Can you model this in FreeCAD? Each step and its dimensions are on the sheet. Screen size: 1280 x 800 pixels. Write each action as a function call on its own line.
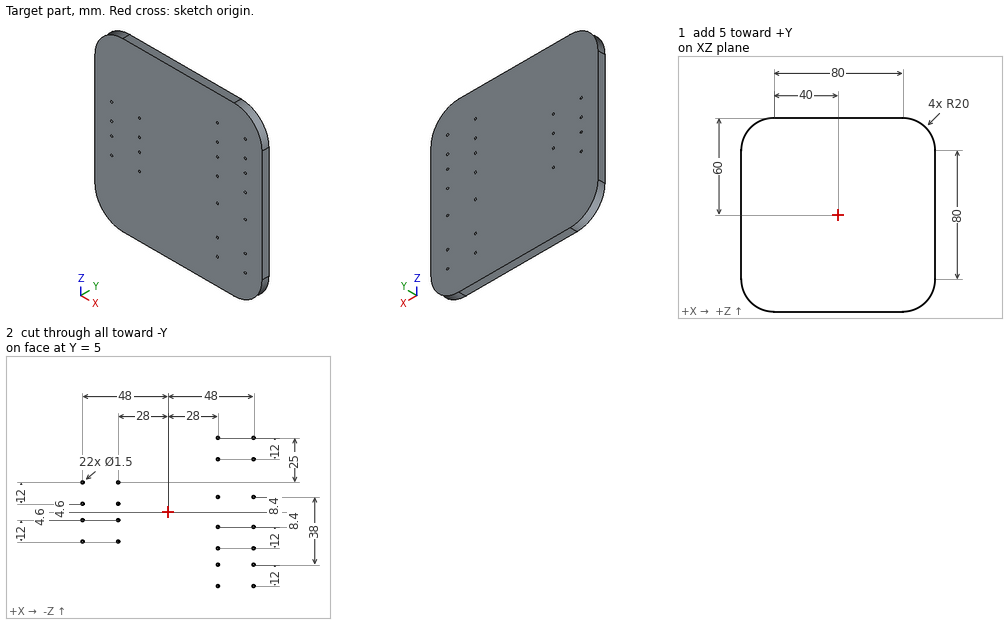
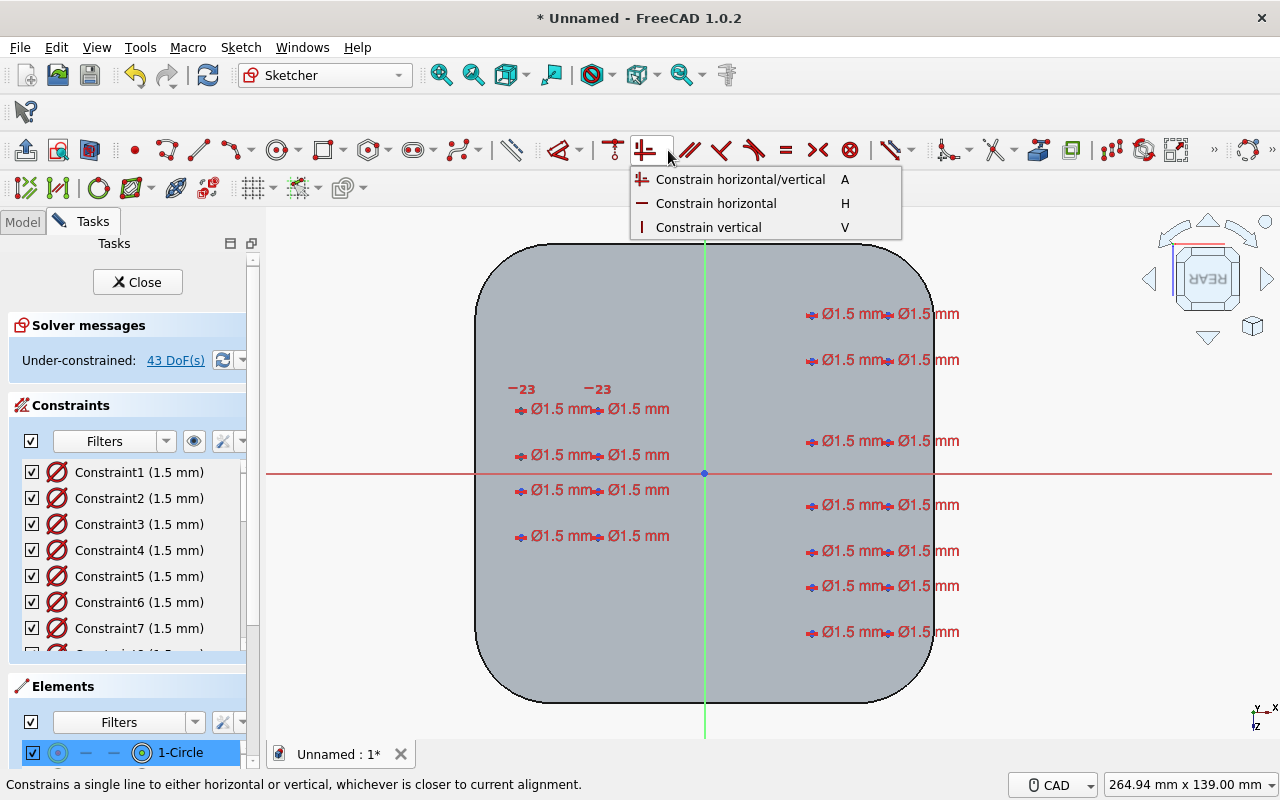
click(766, 227)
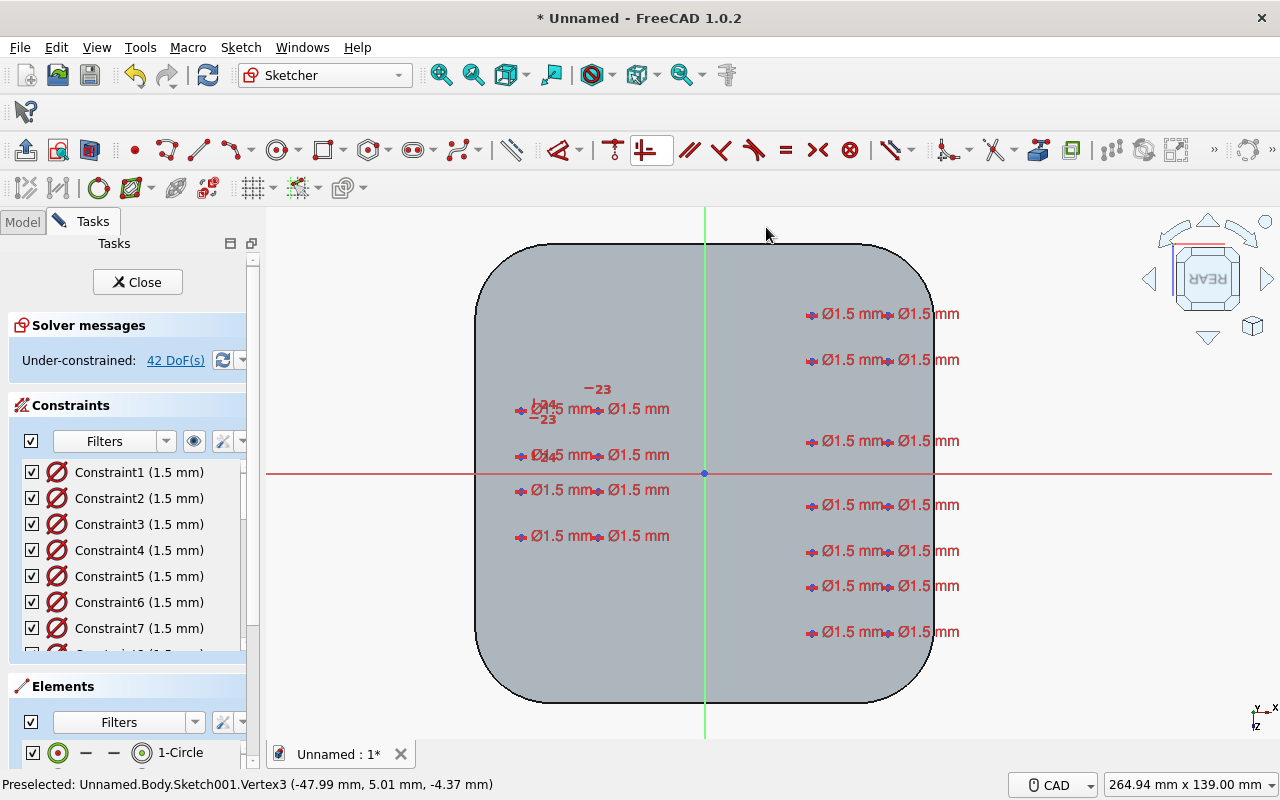
click(598, 411)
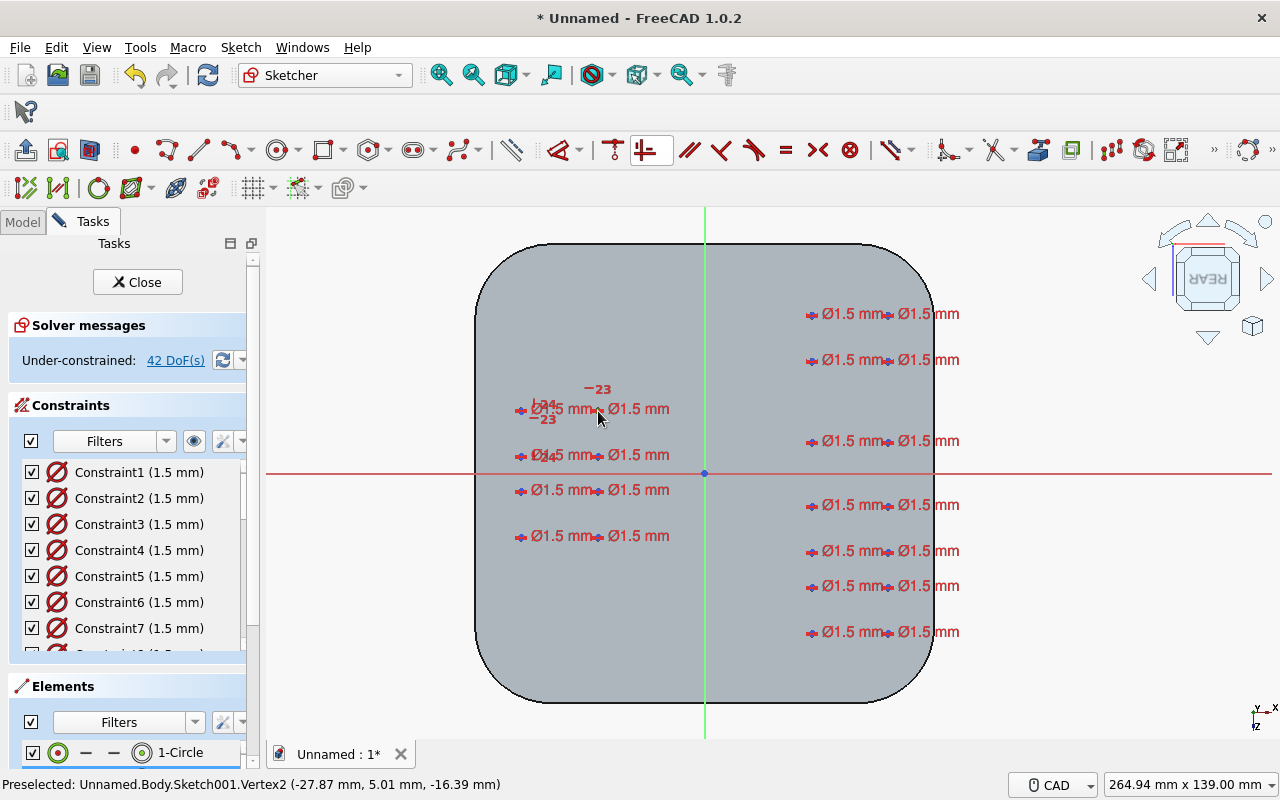
click(598, 457)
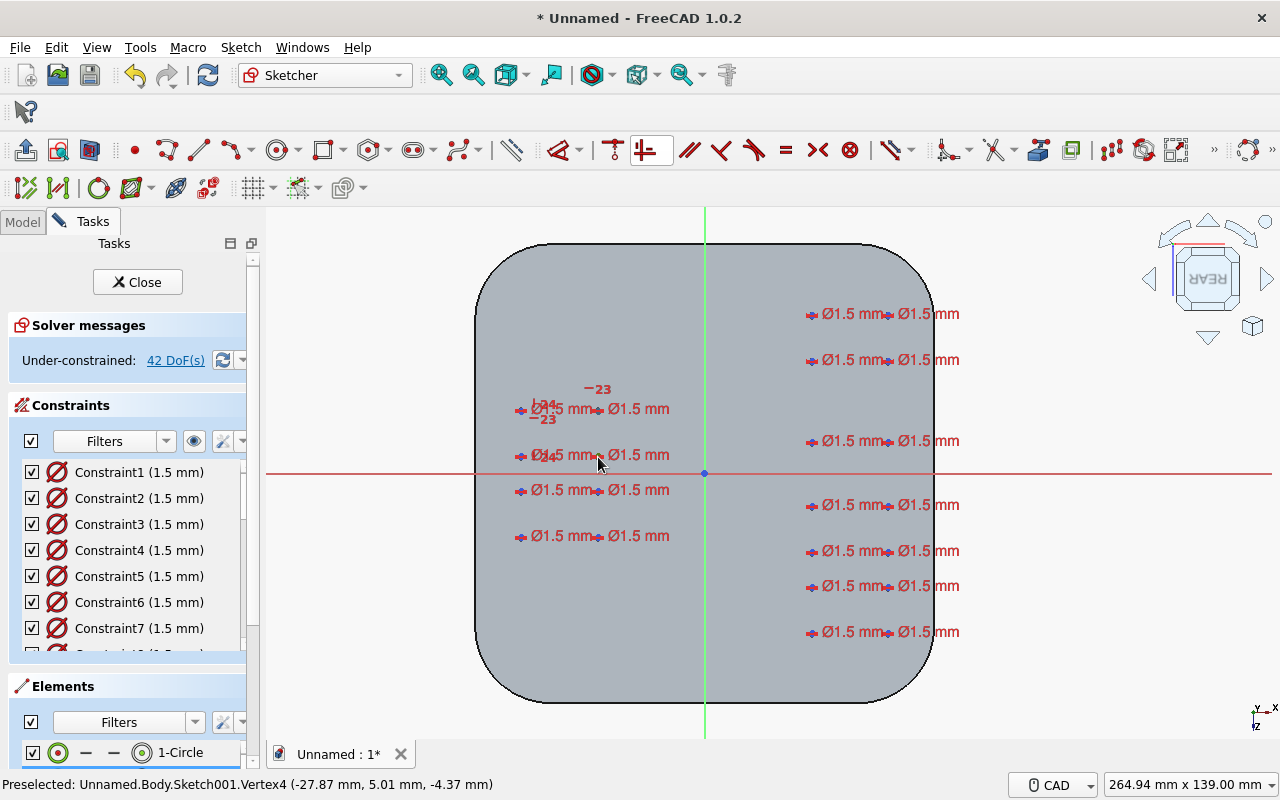
key(v)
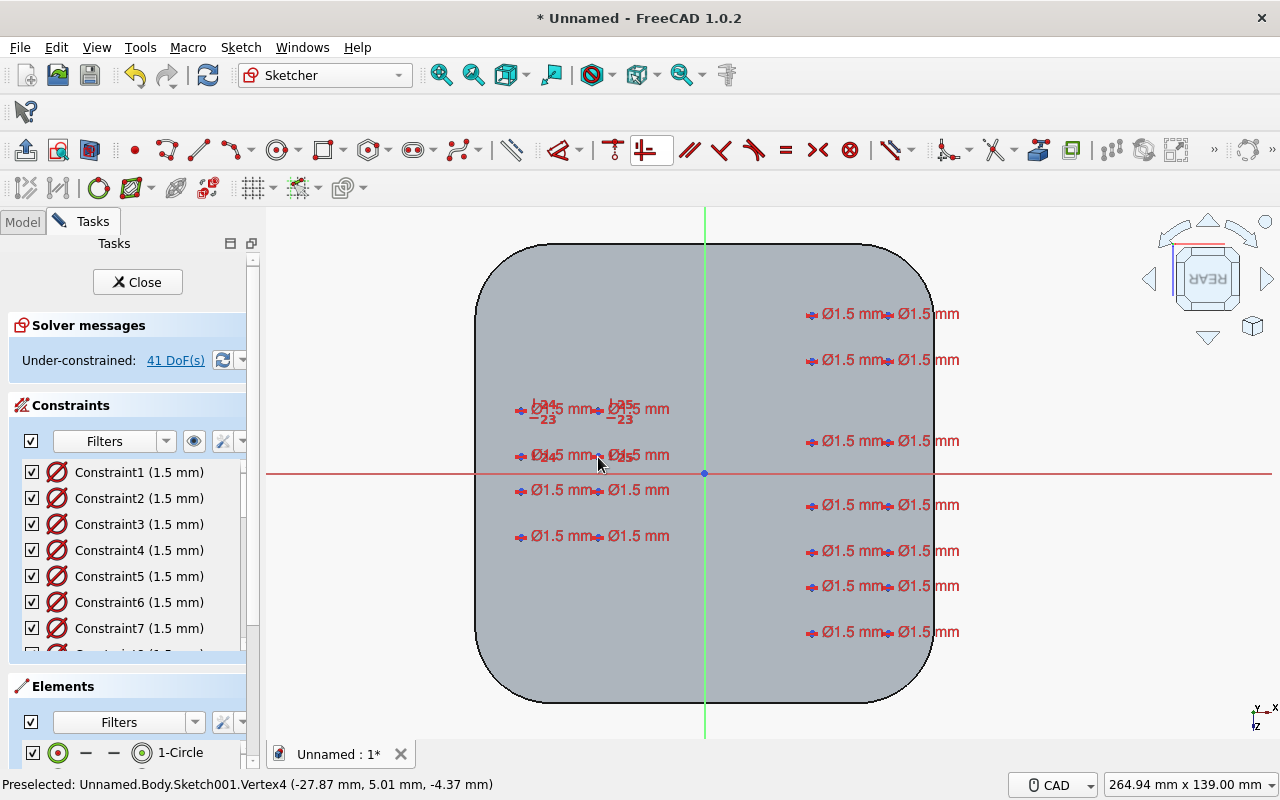
click(521, 457)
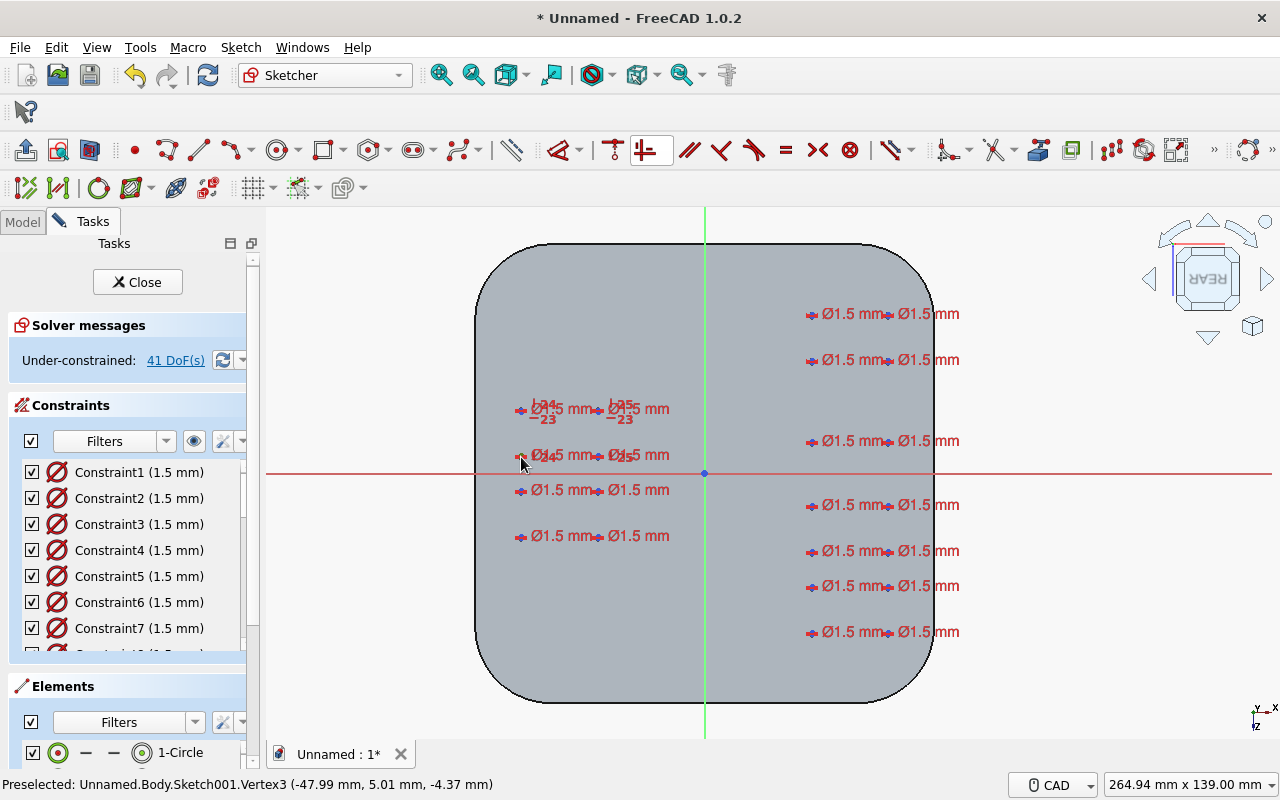
click(598, 457)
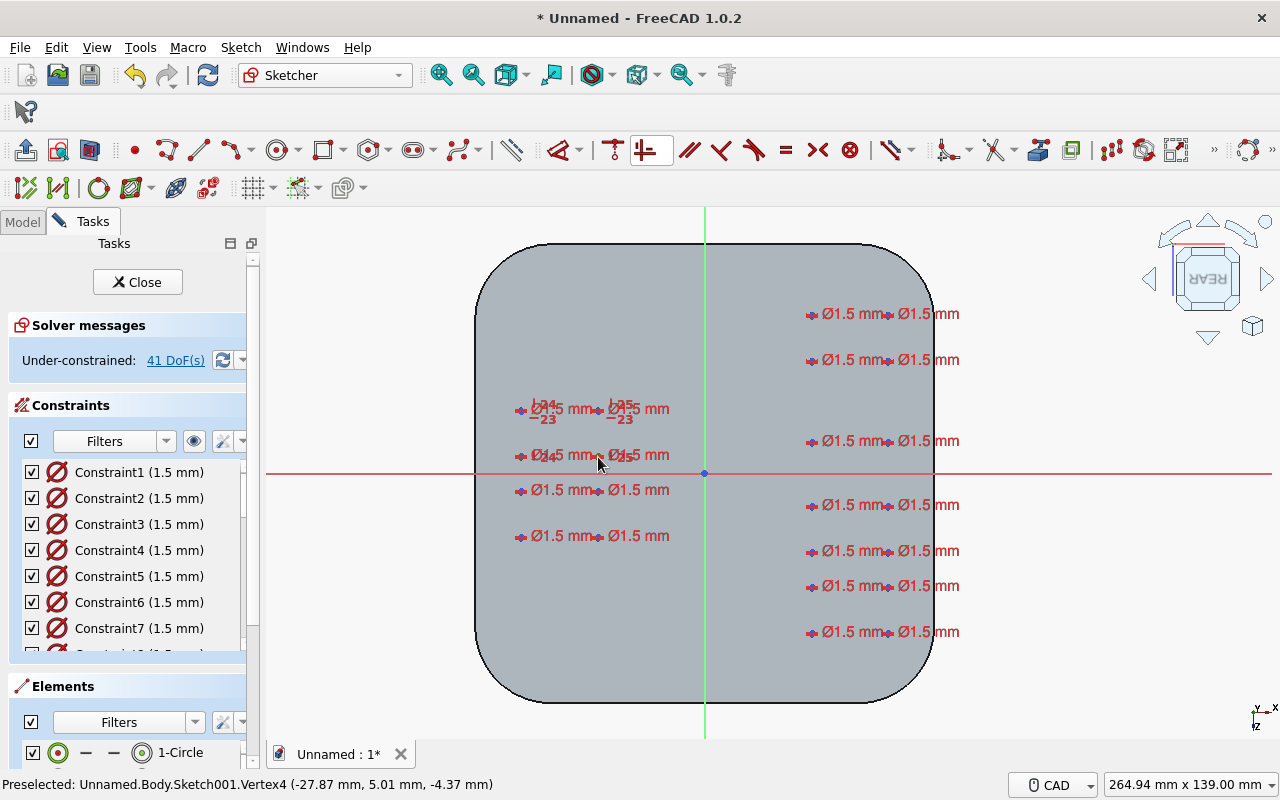
click(668, 150)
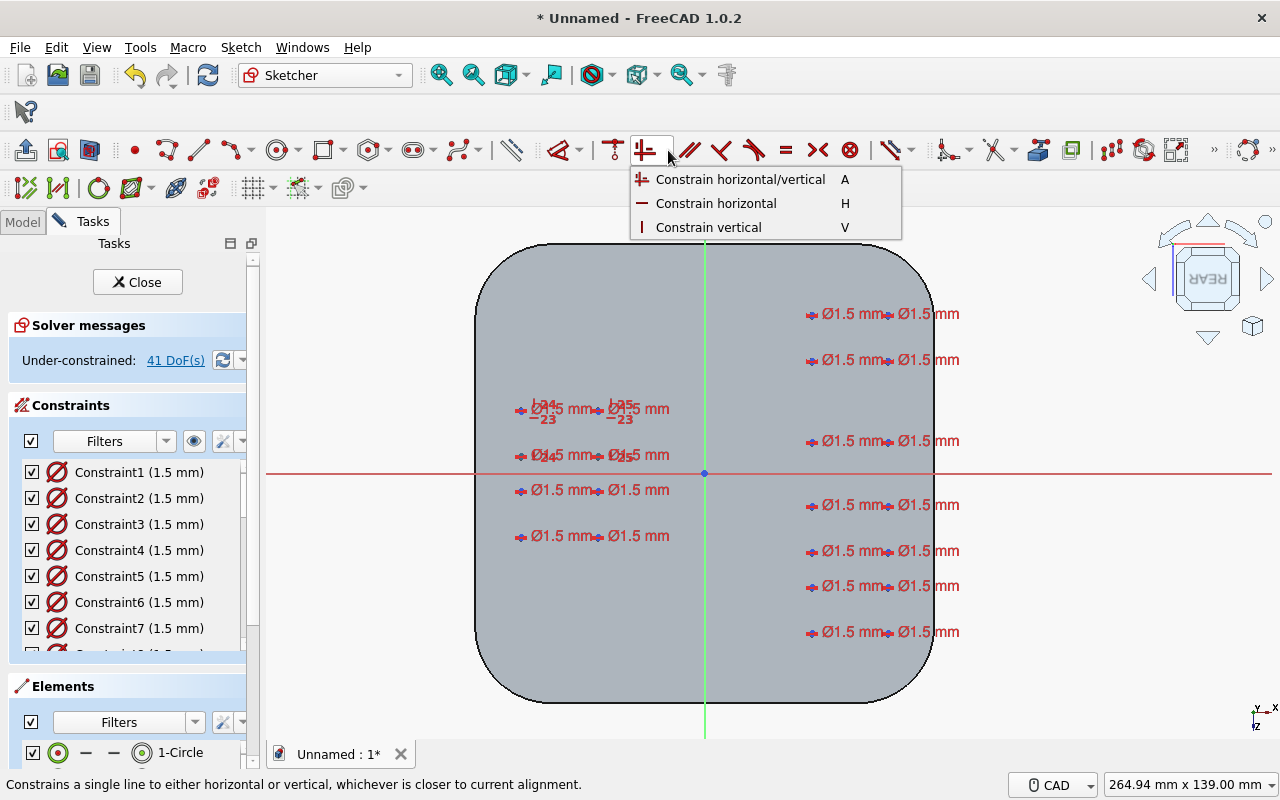
click(766, 203)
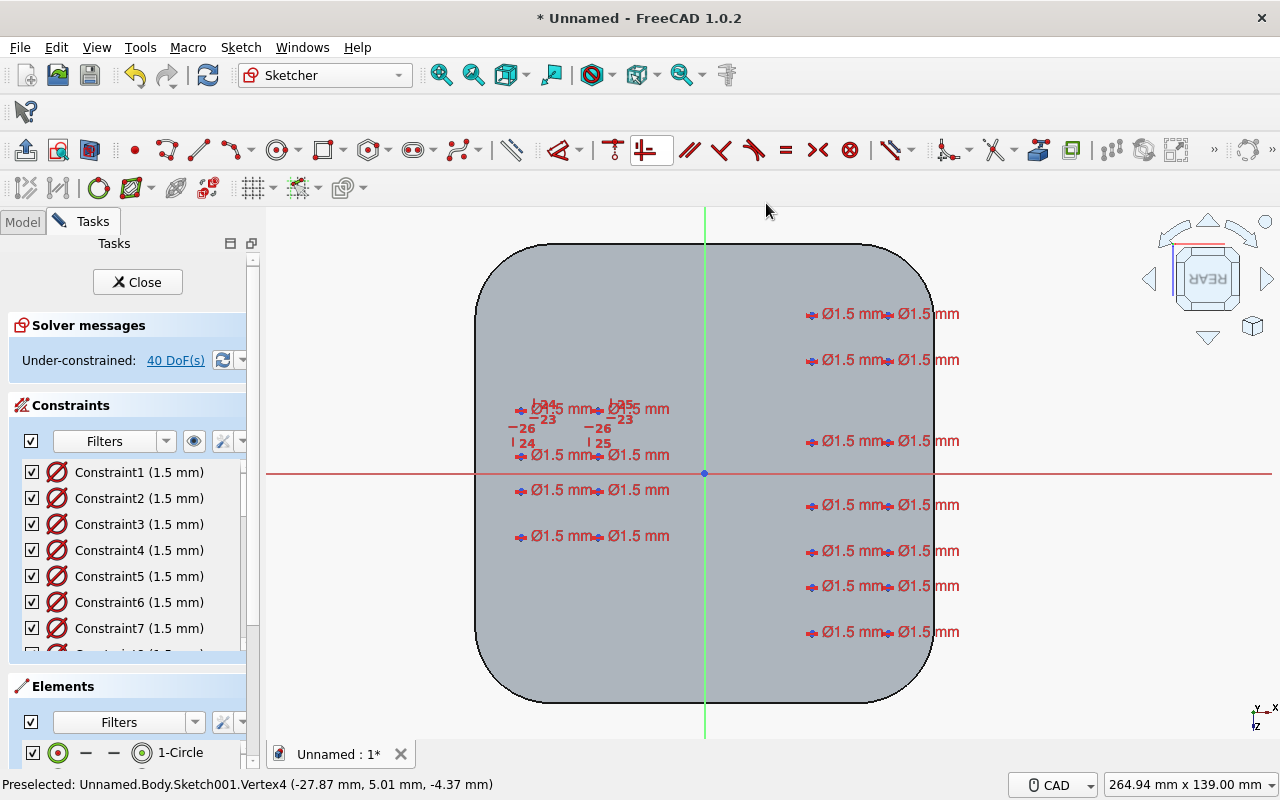
click(598, 457)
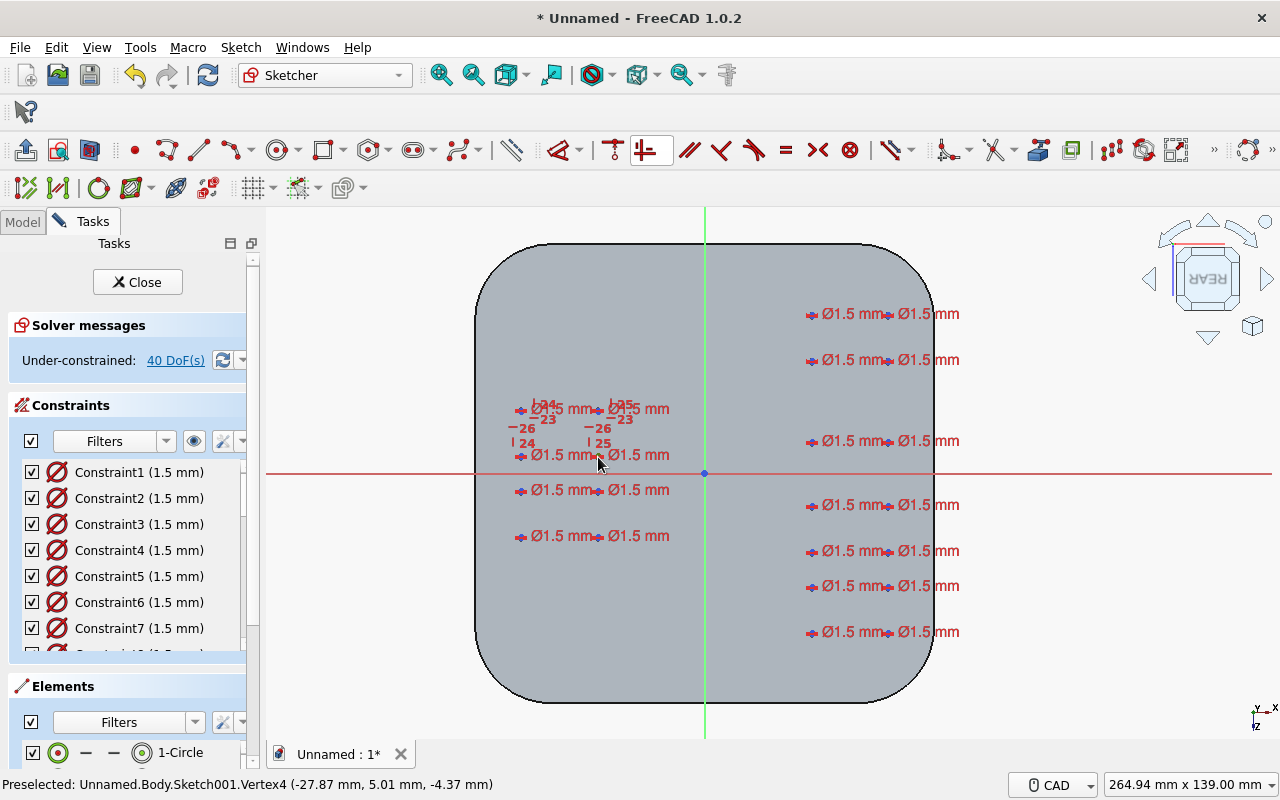
click(598, 492)